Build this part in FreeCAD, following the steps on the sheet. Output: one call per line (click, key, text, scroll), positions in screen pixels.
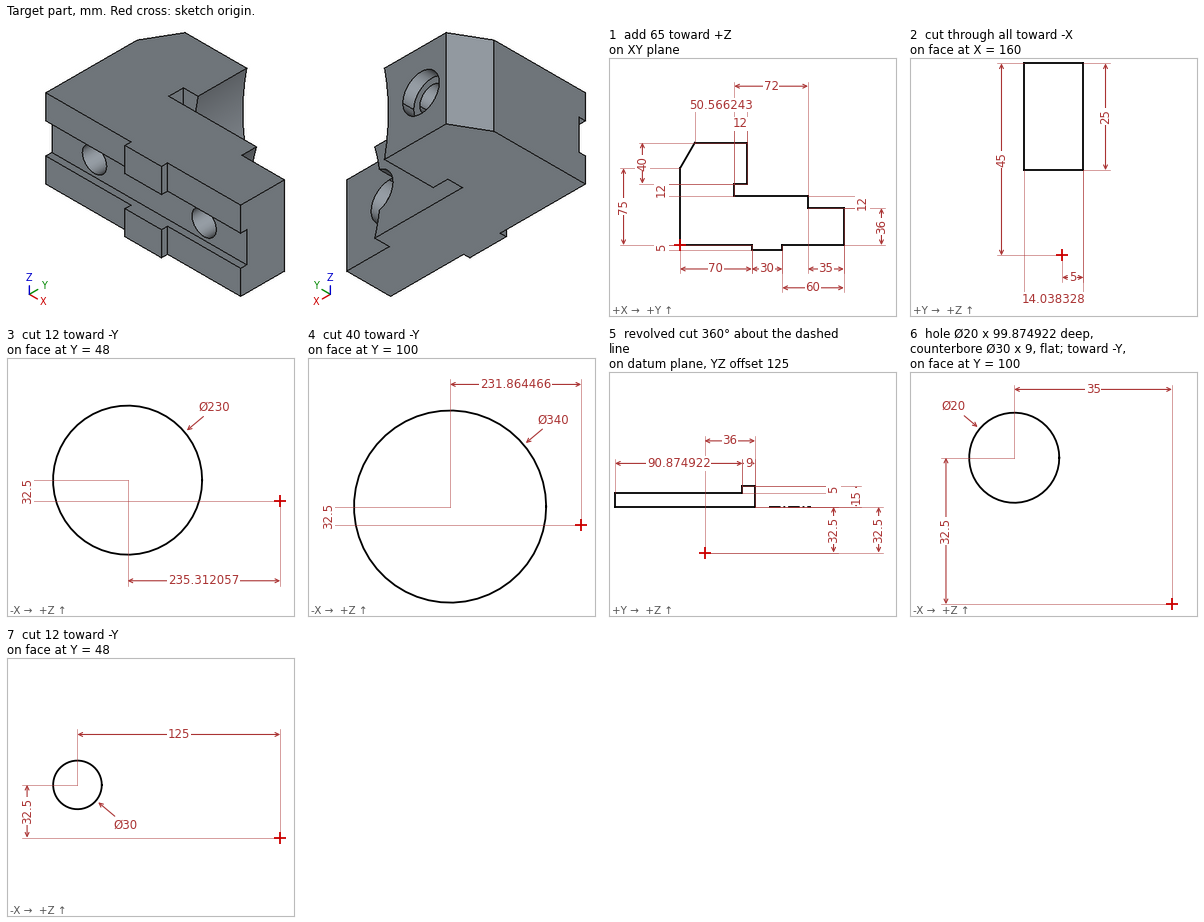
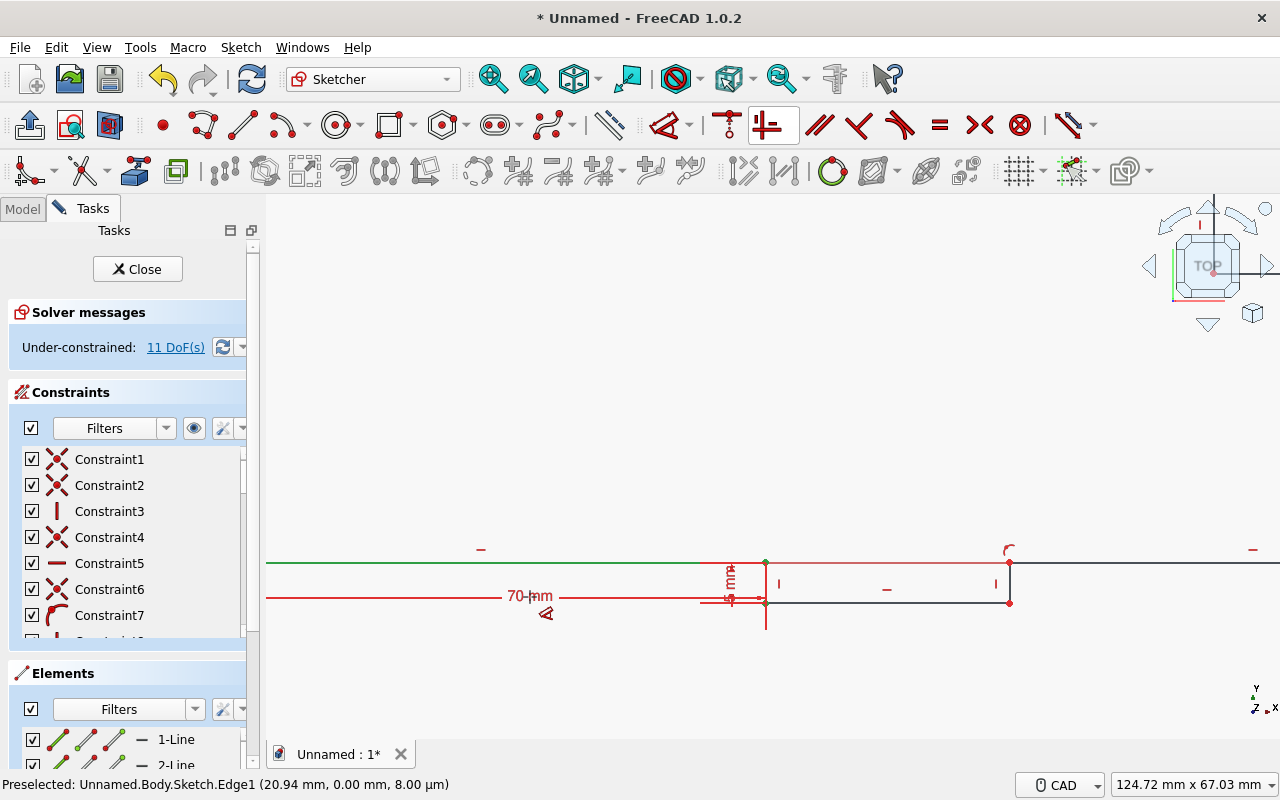
click(839, 603)
click(888, 637)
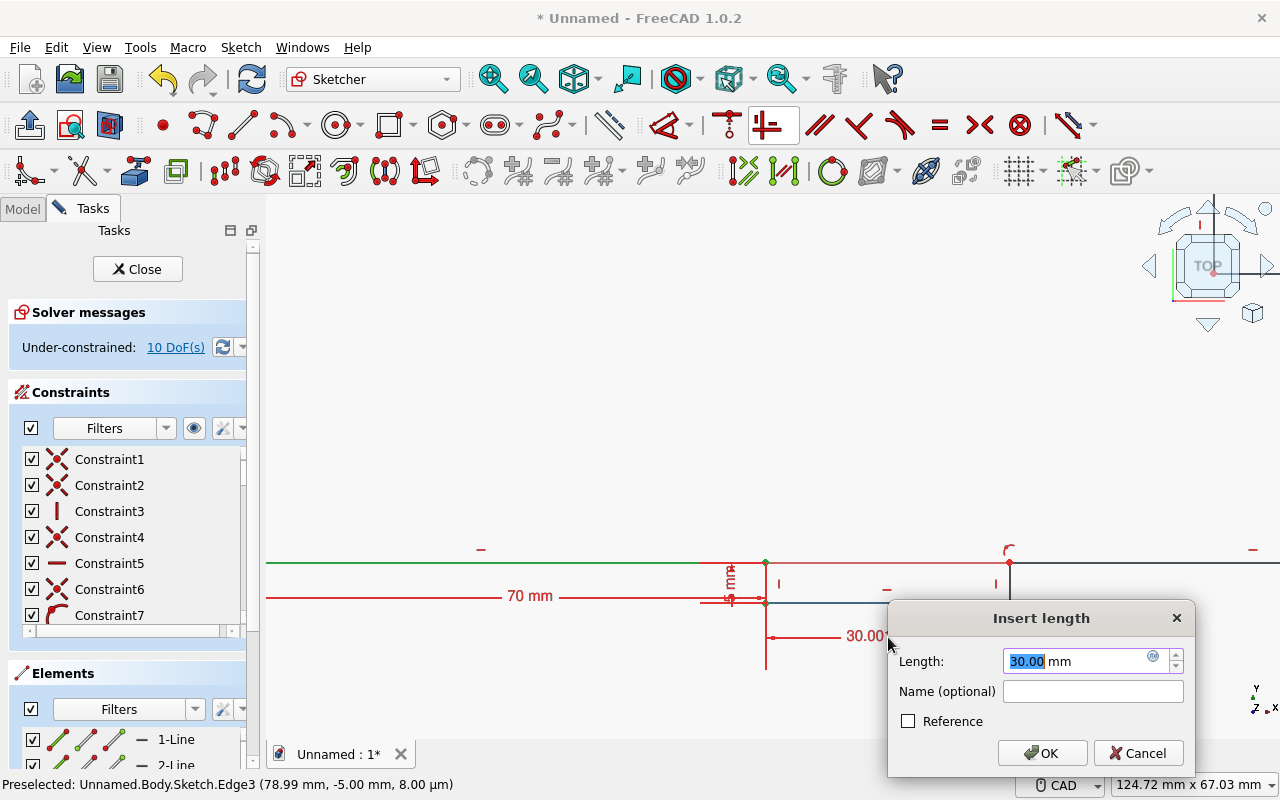
text(30)
key(Return)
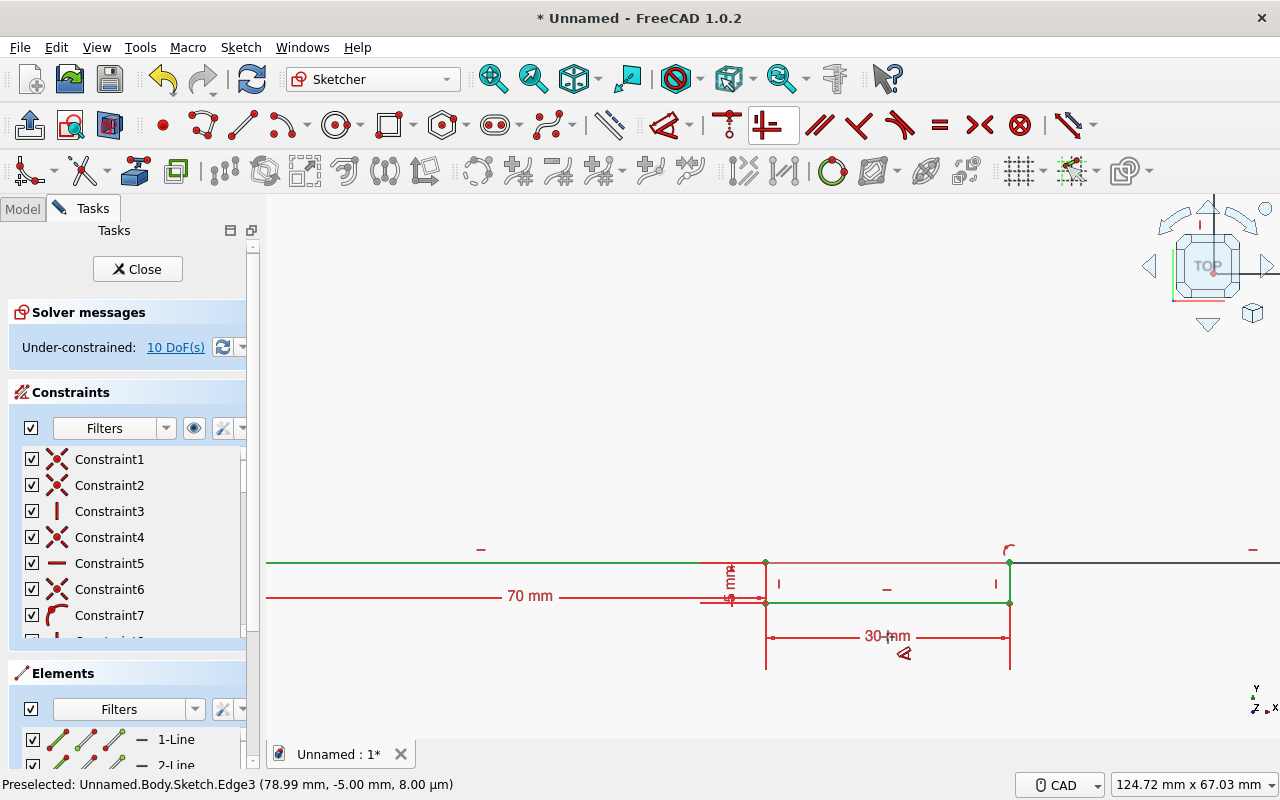
click(1107, 563)
click(1062, 597)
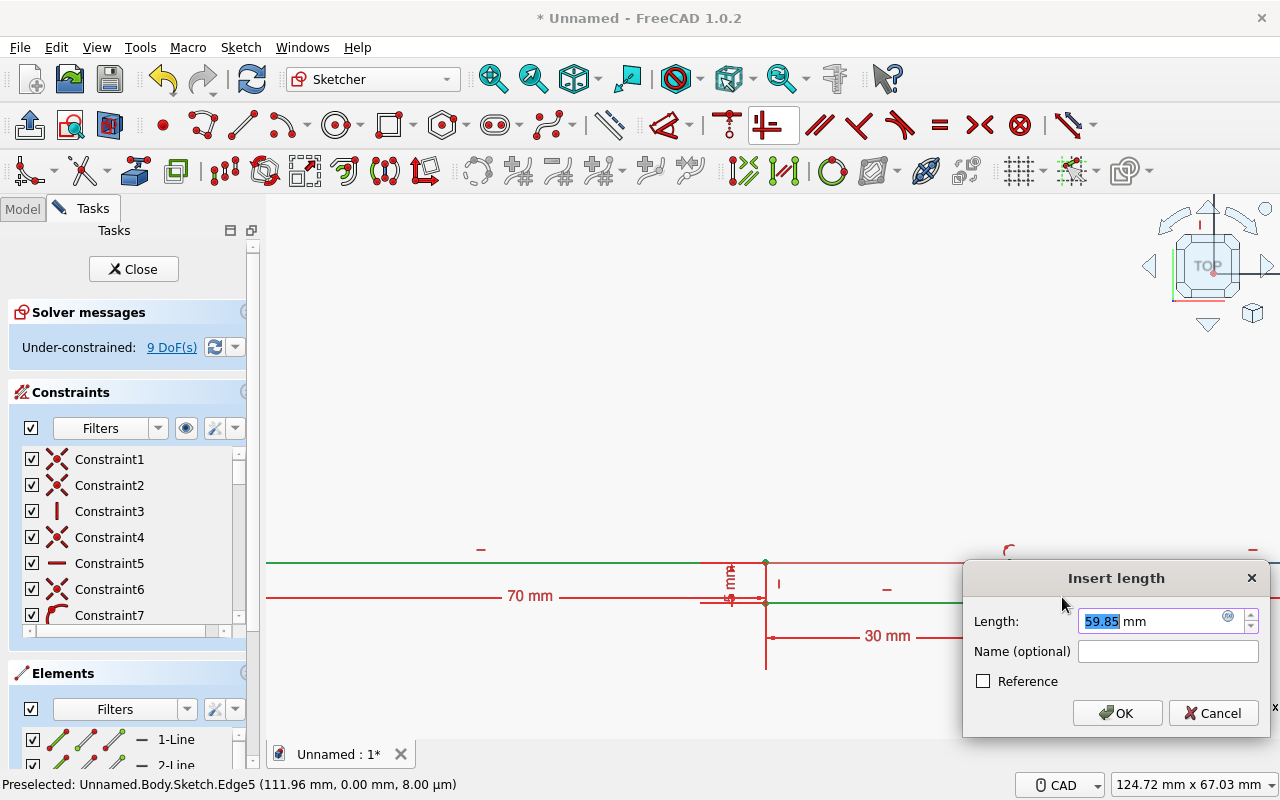
text(60)
key(Return)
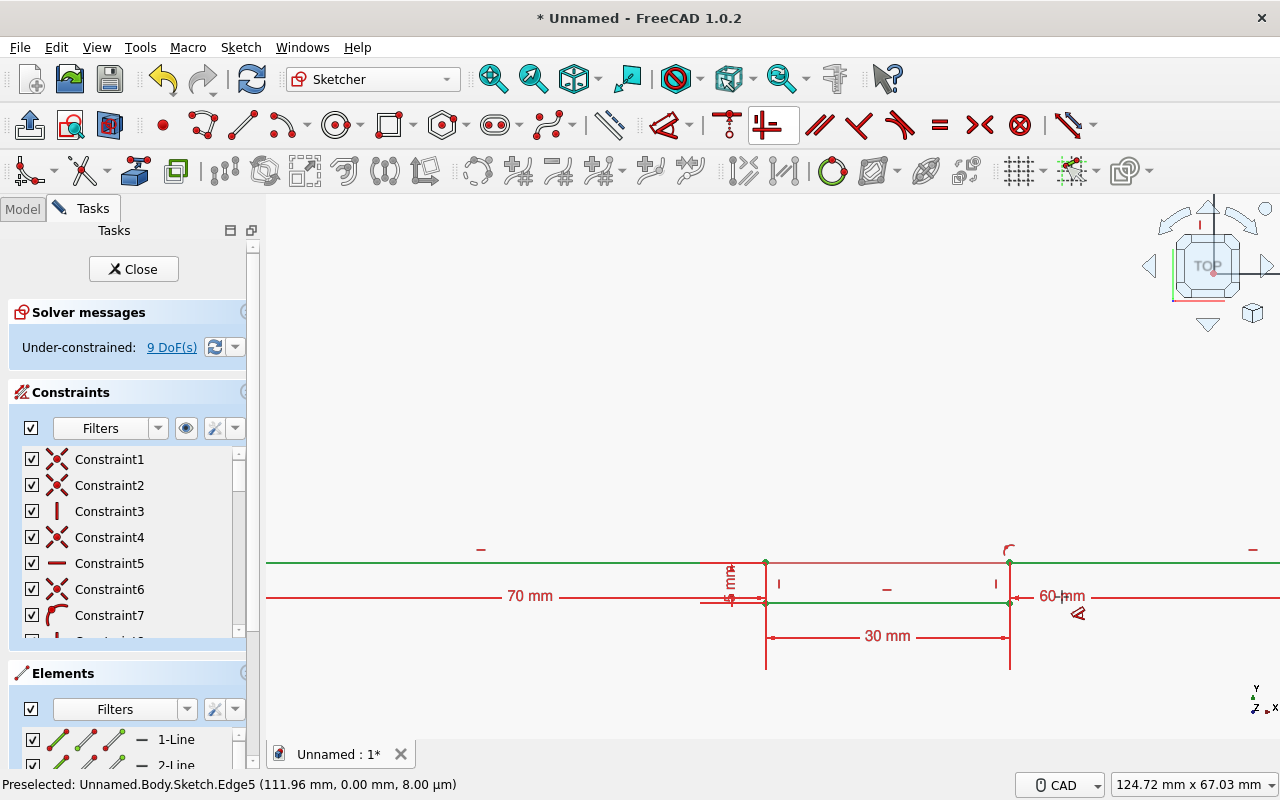
scroll(621, 635, down, 5)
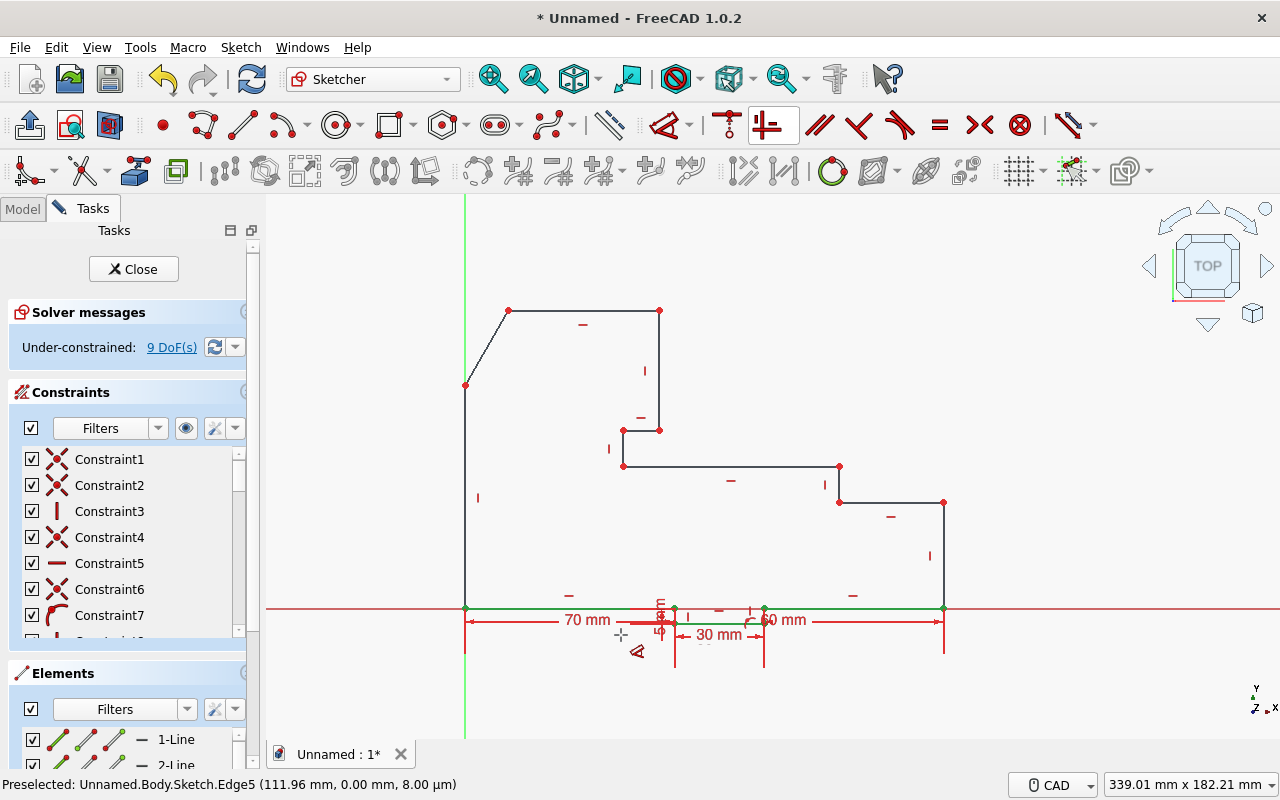
click(944, 577)
click(978, 556)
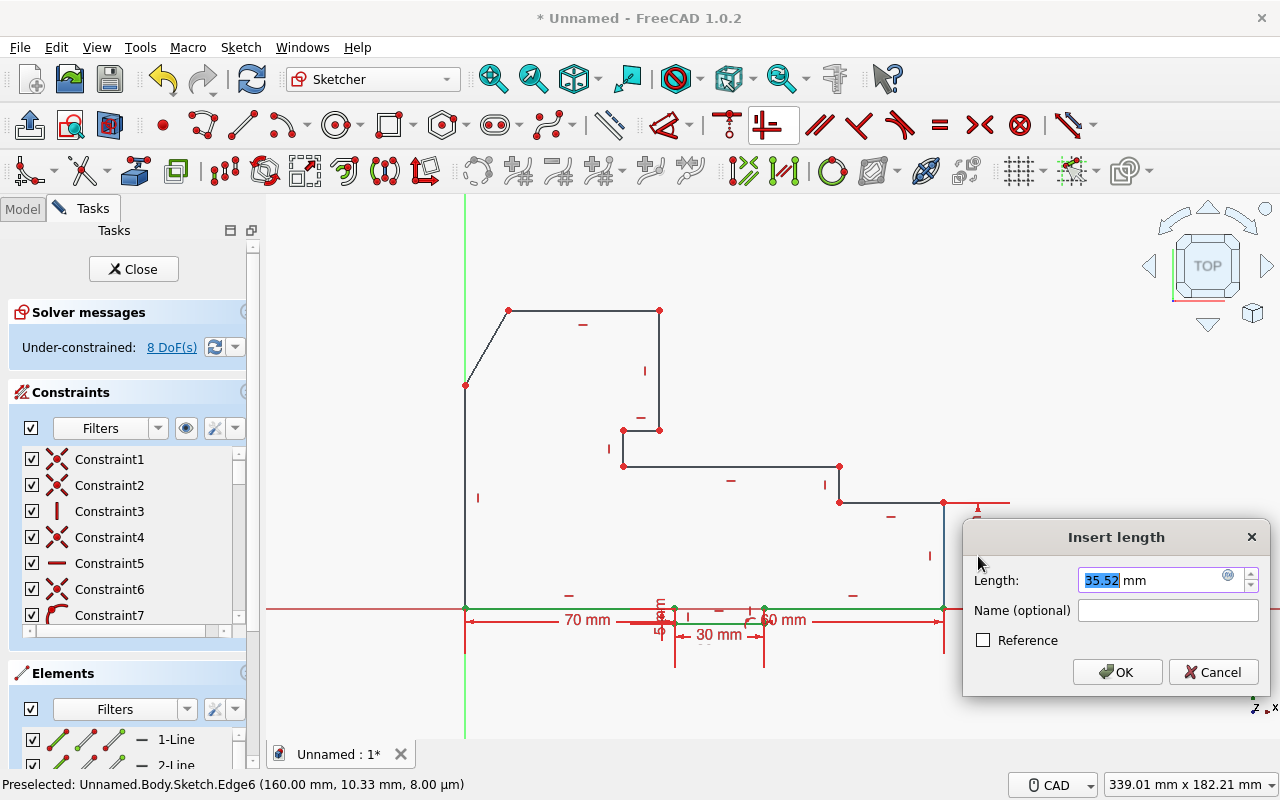
text(36)
key(Return)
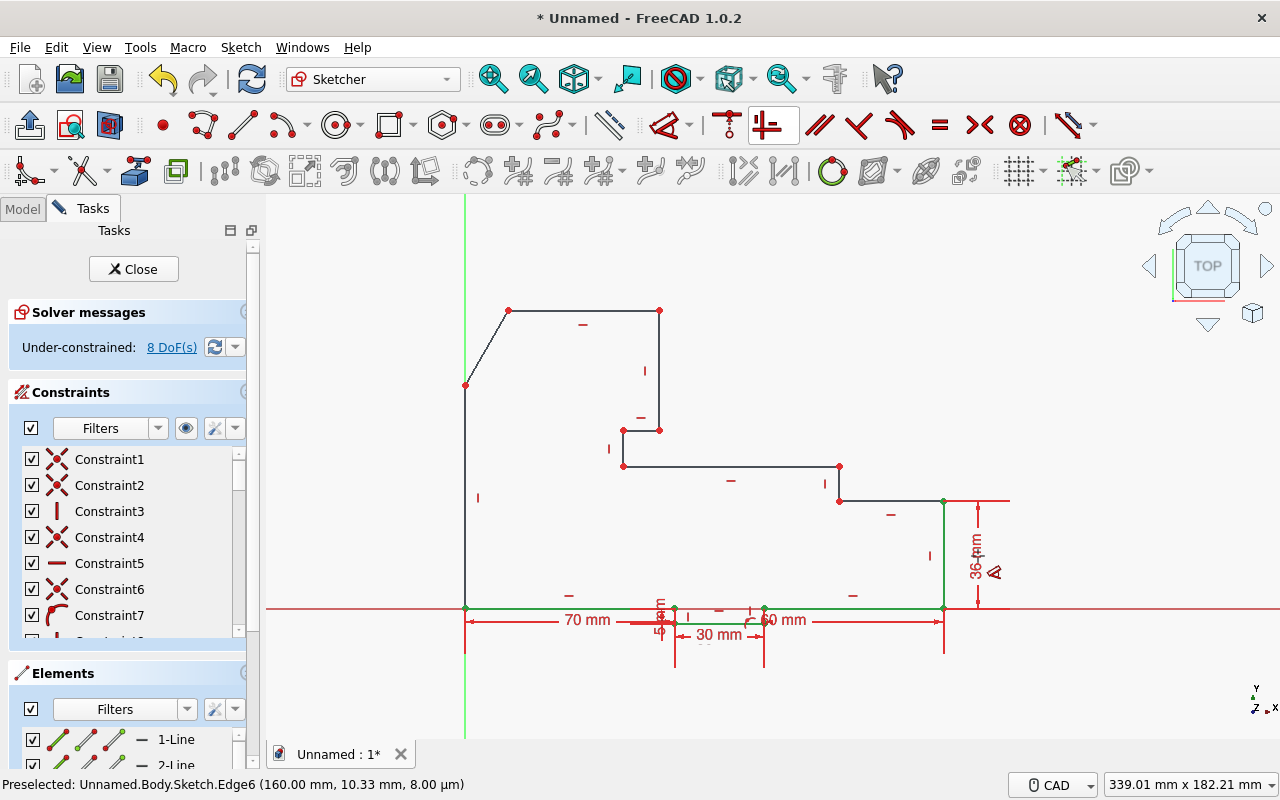
click(912, 501)
click(891, 535)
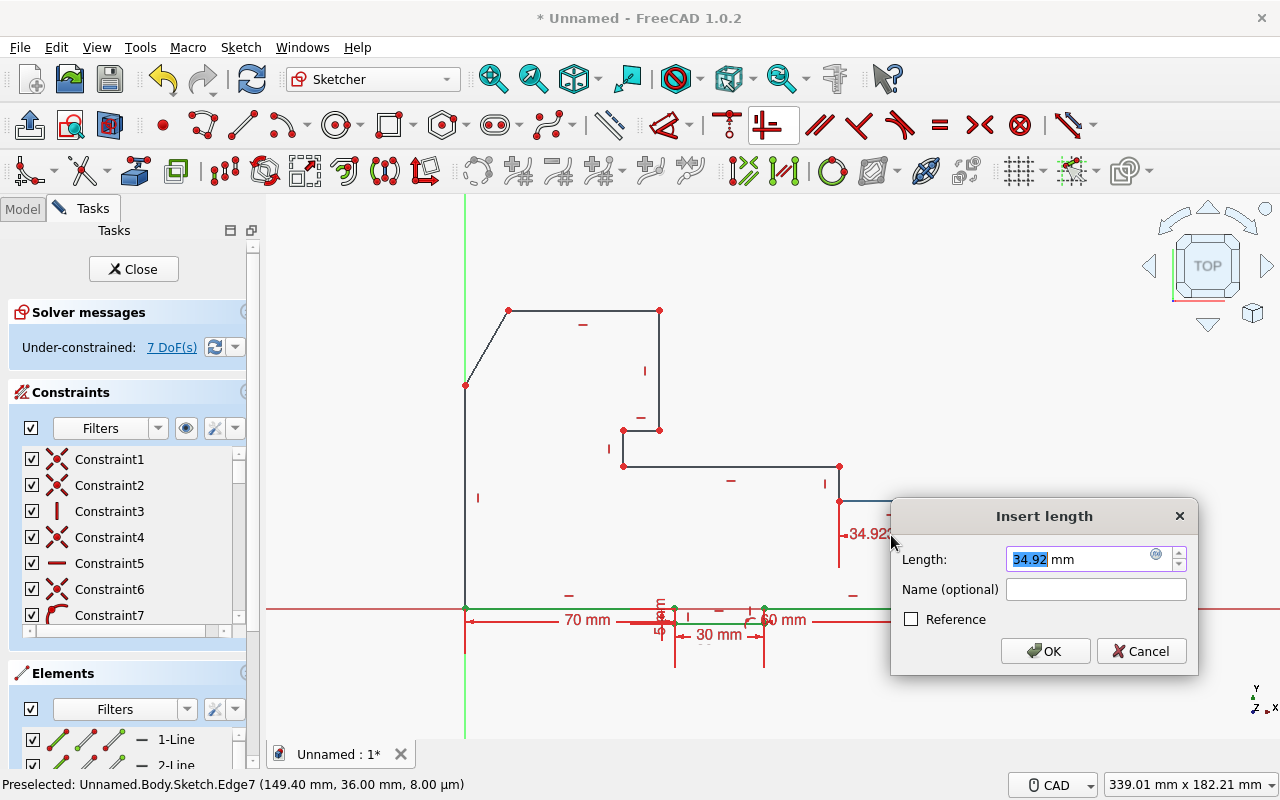
text(35)
key(Return)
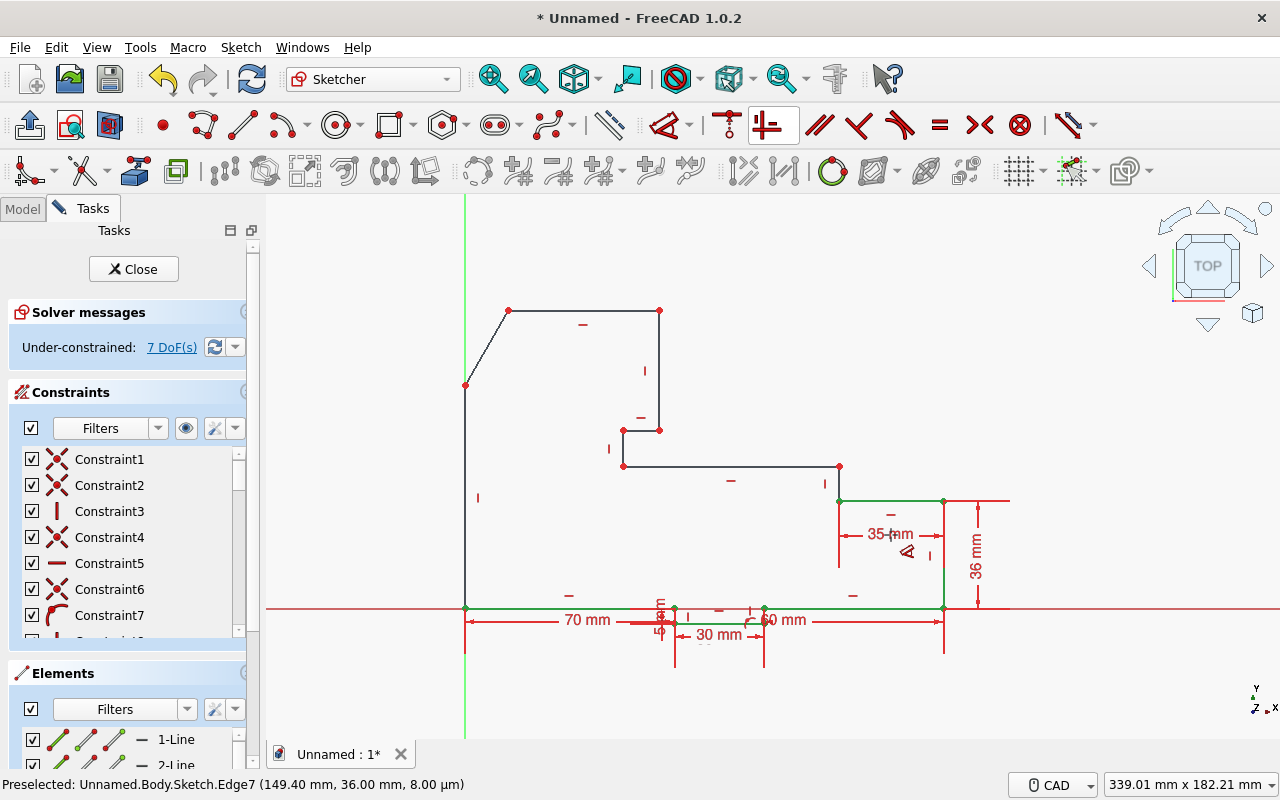
scroll(839, 491, up, 2)